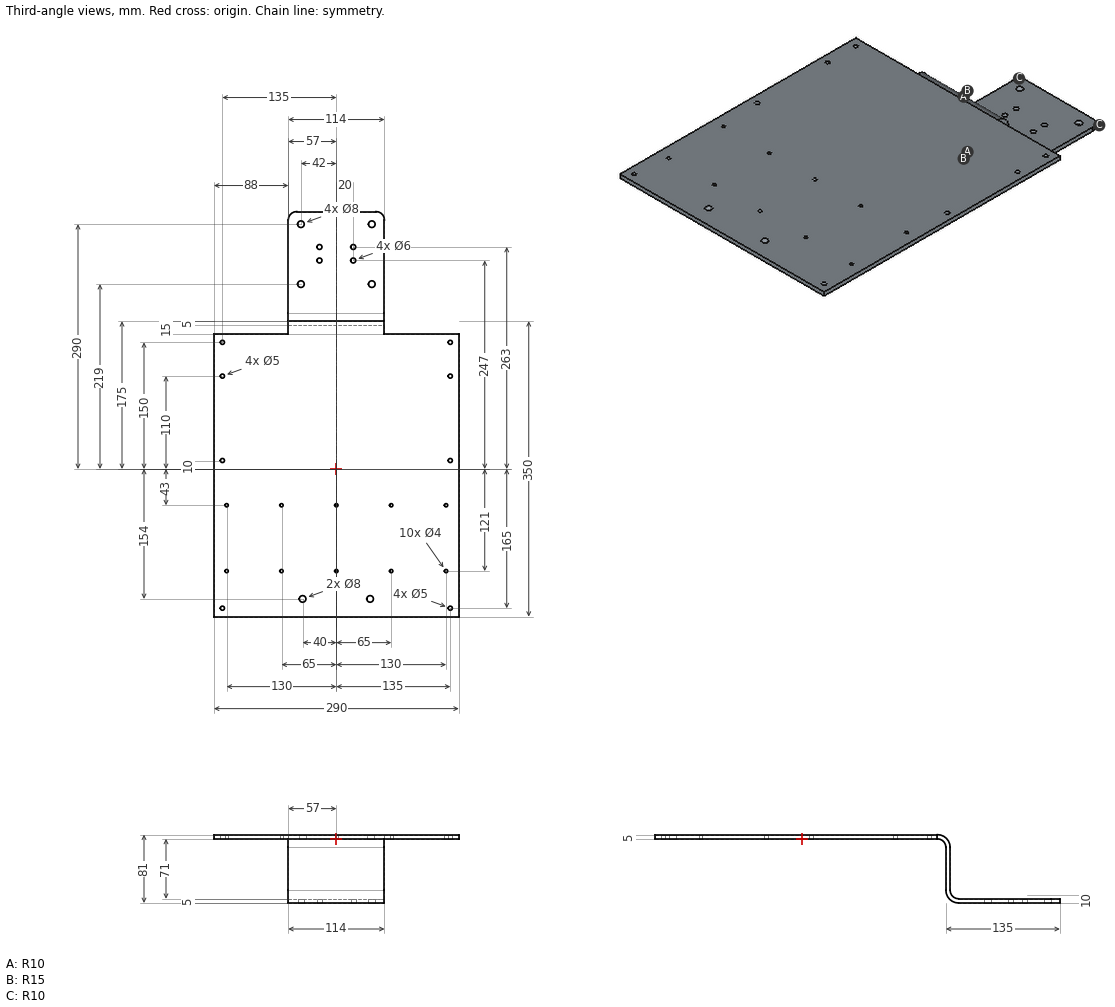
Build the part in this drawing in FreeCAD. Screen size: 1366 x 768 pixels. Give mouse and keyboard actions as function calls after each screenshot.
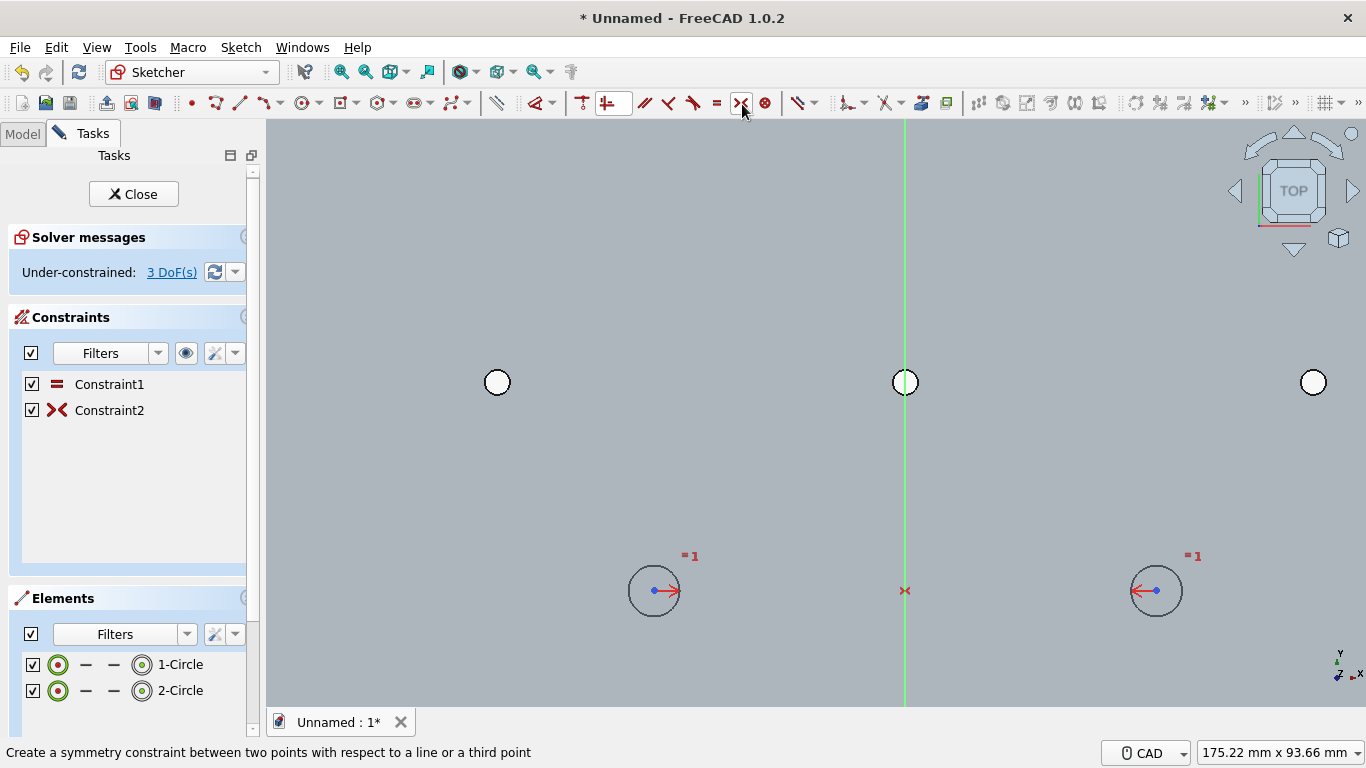
click(536, 104)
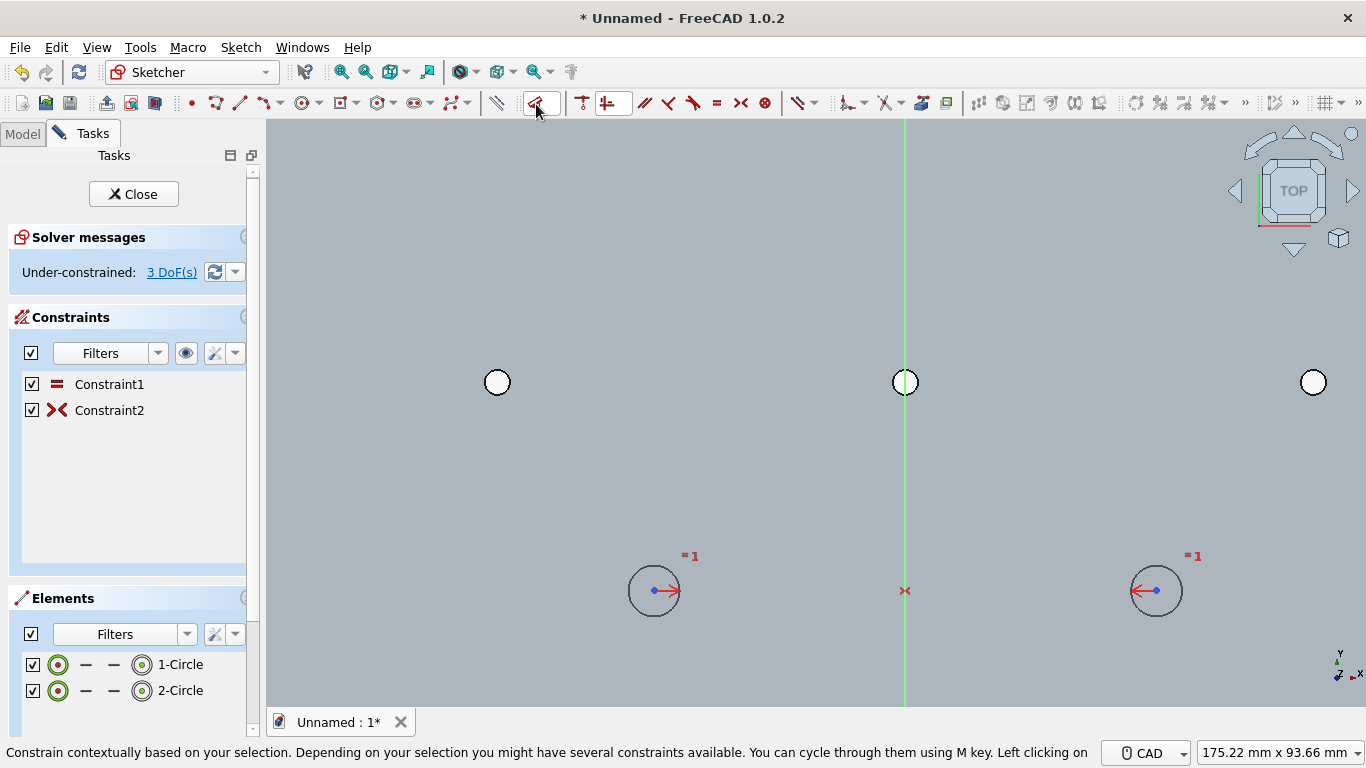
click(672, 573)
click(695, 550)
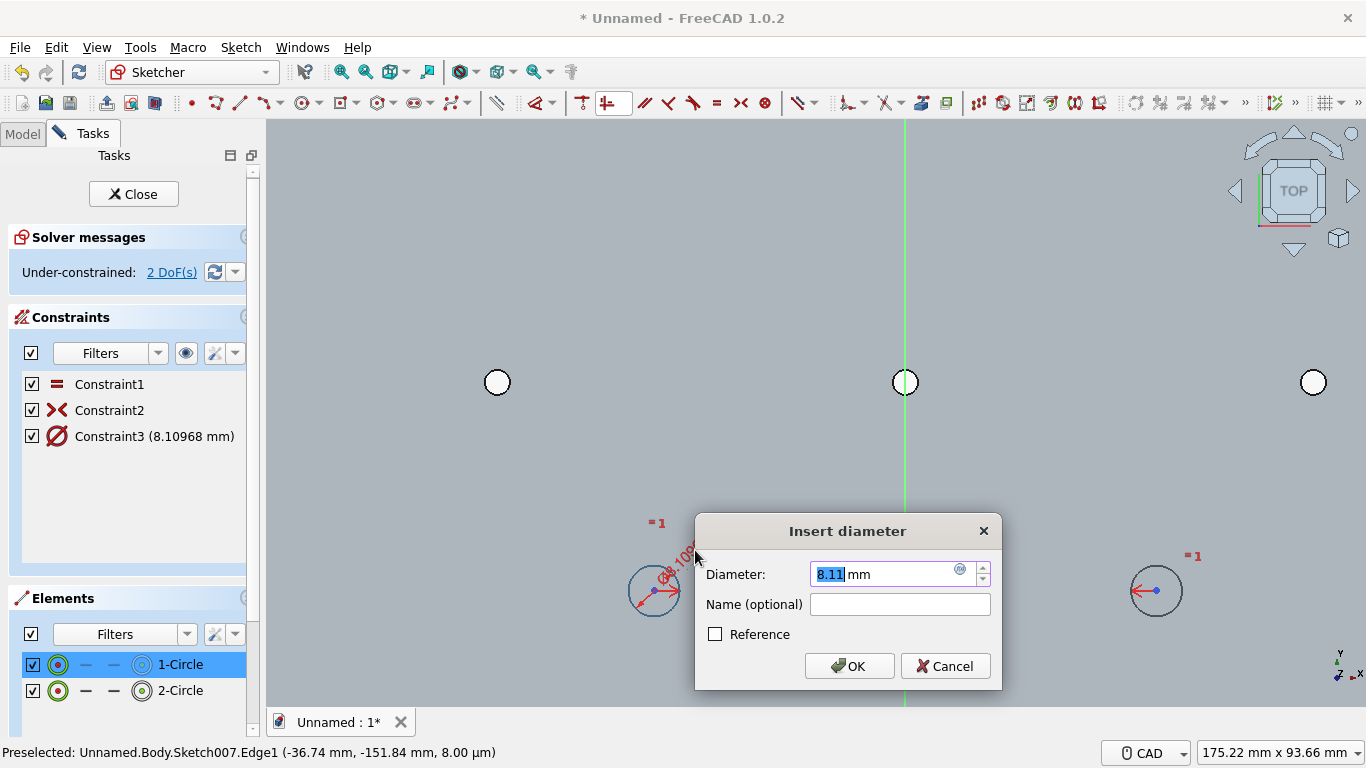
text(8)
key(Return)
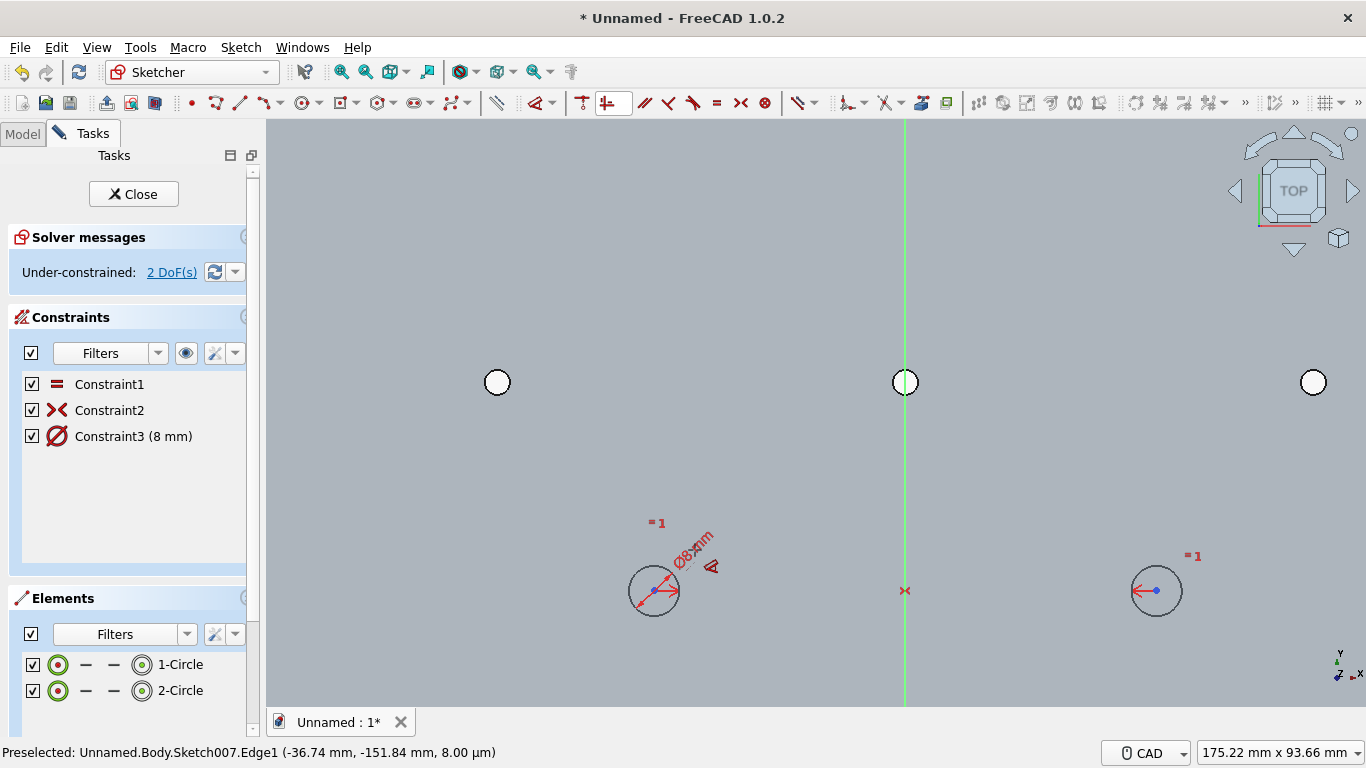
click(654, 591)
click(780, 625)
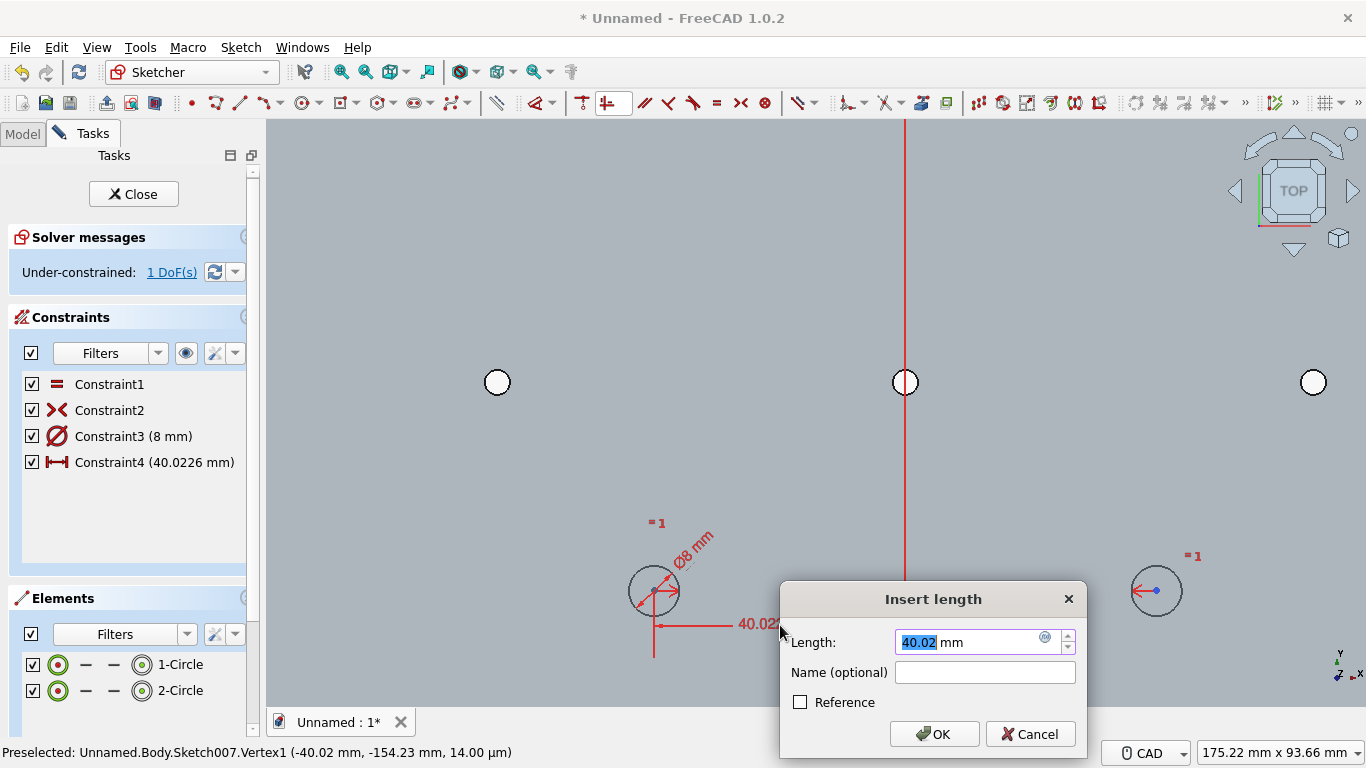
text(40)
key(Return)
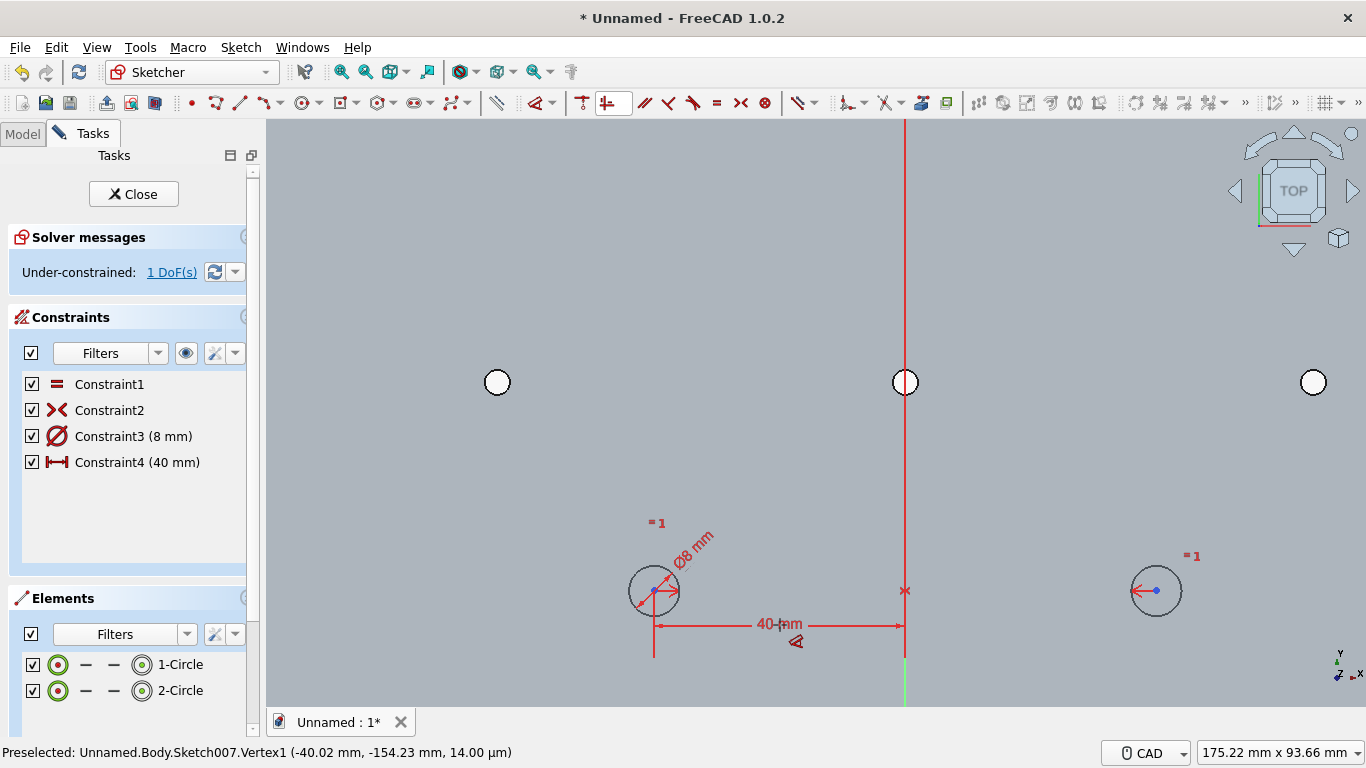
click(654, 591)
click(620, 369)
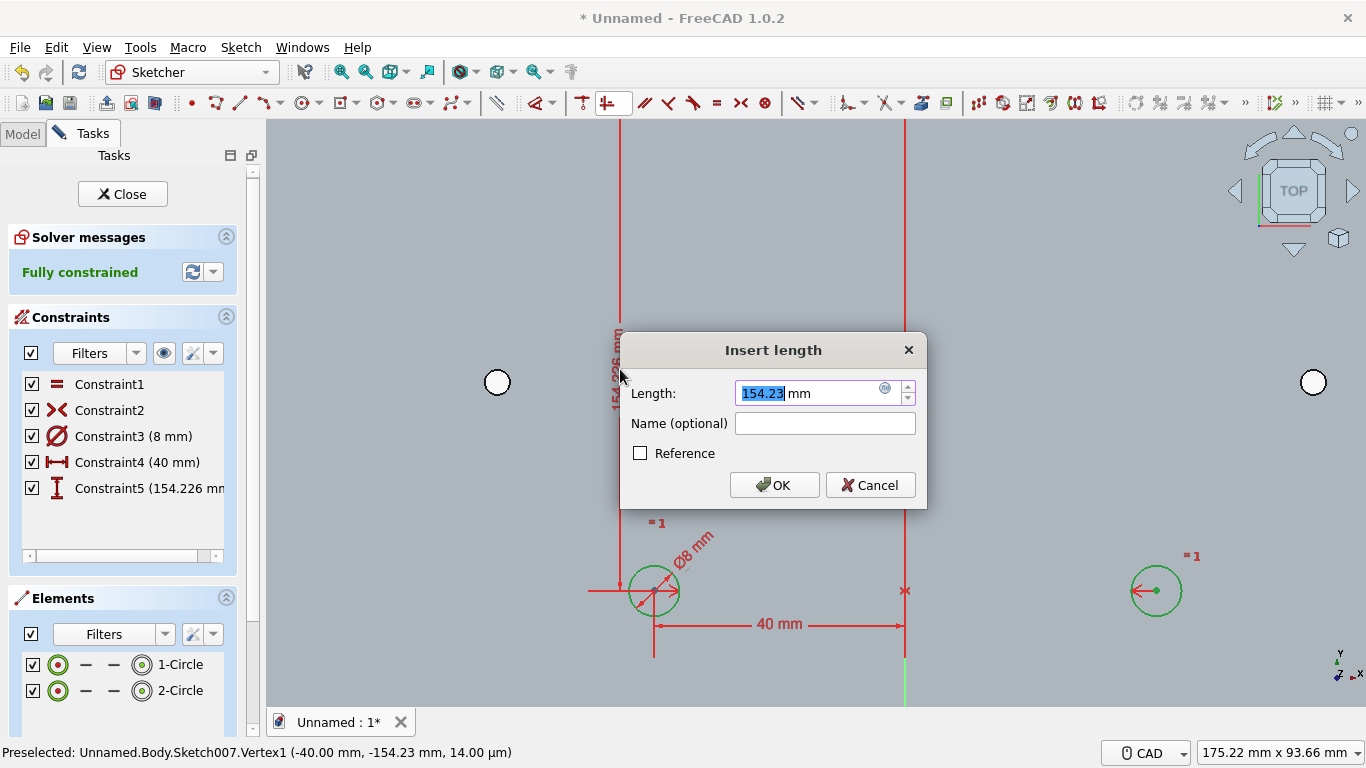
text(154)
key(Return)
key(Escape)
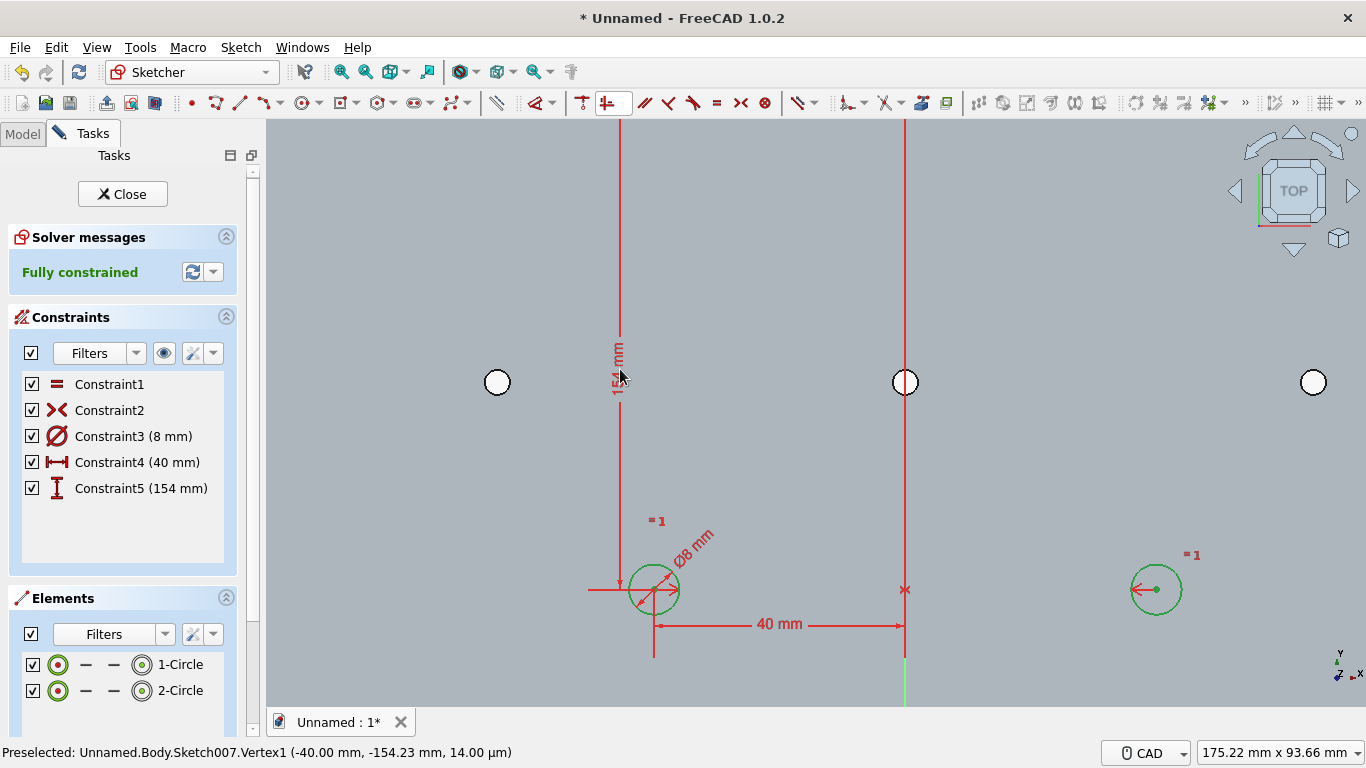
click(123, 194)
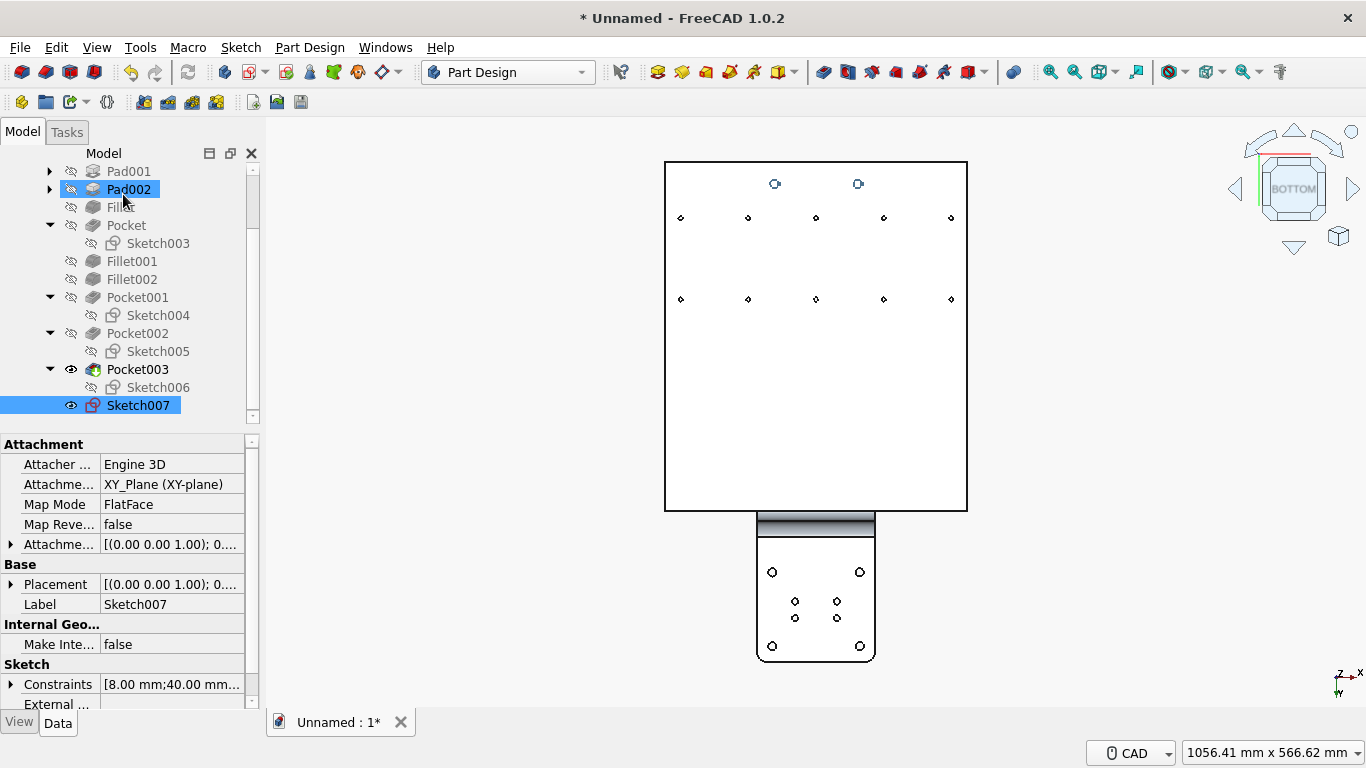
click(824, 72)